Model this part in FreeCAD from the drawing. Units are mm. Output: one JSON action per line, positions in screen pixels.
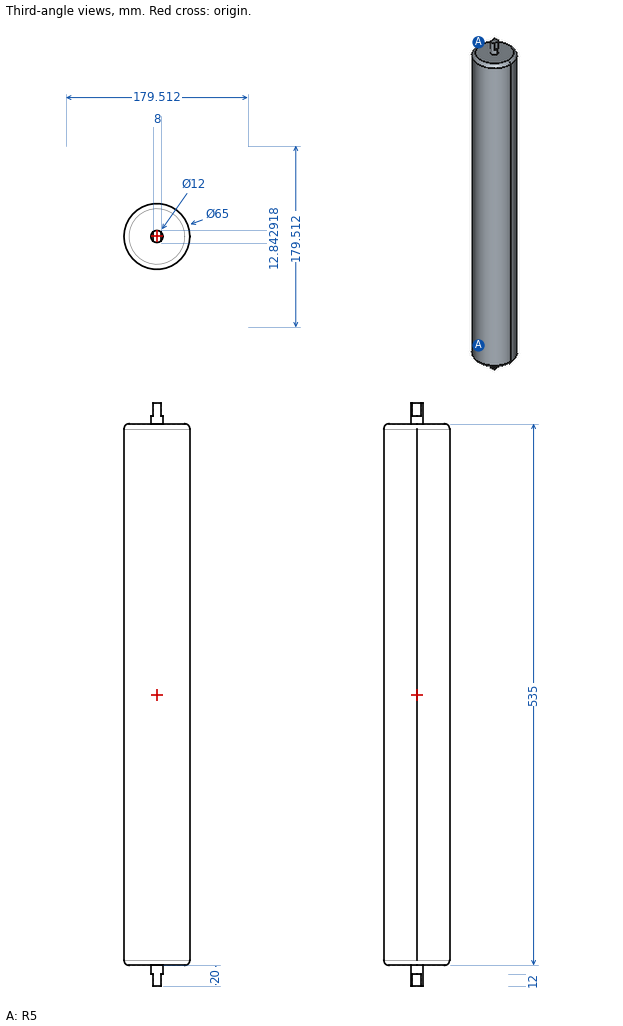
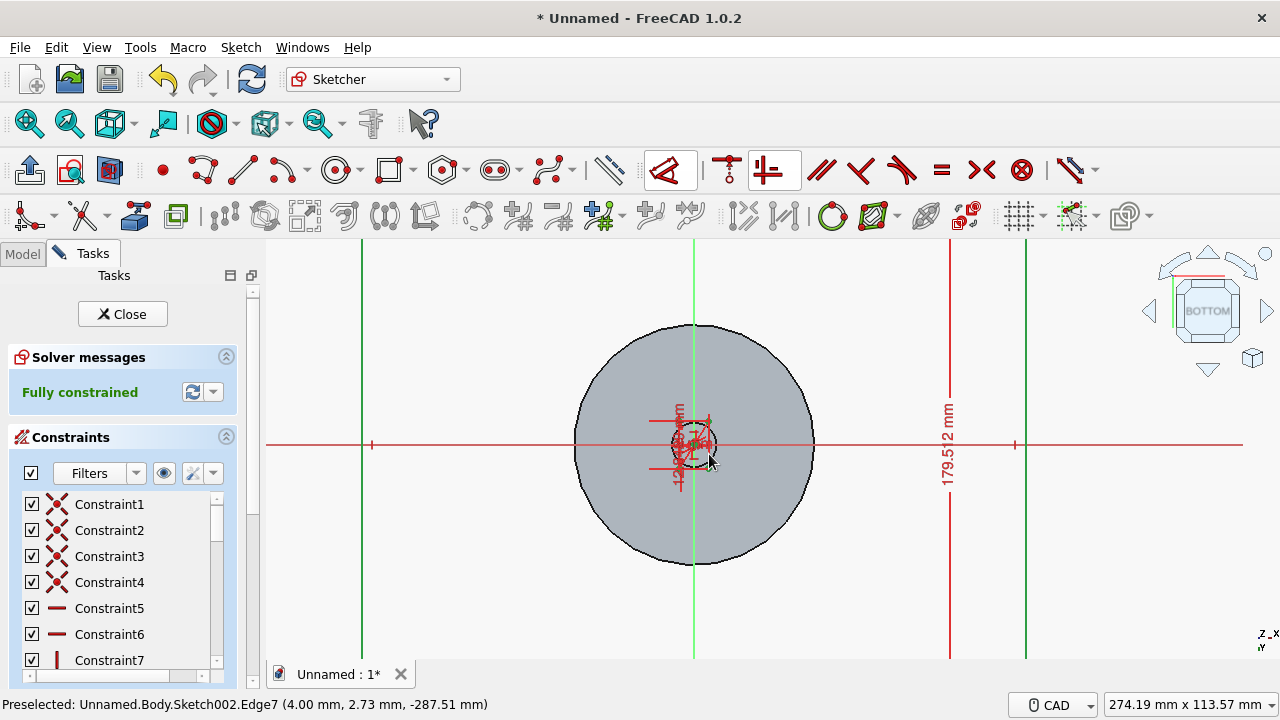
{"action": "left_click", "coordinate": [123, 314]}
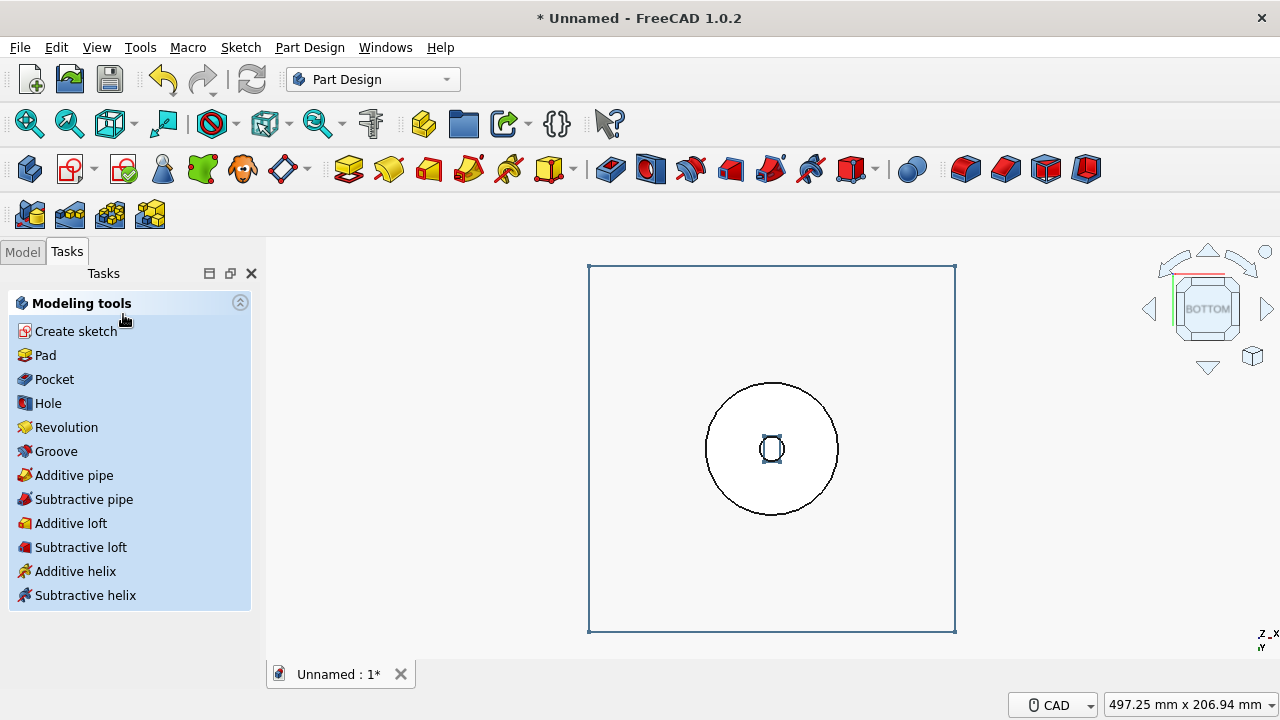
{"action": "left_click", "coordinate": [612, 170]}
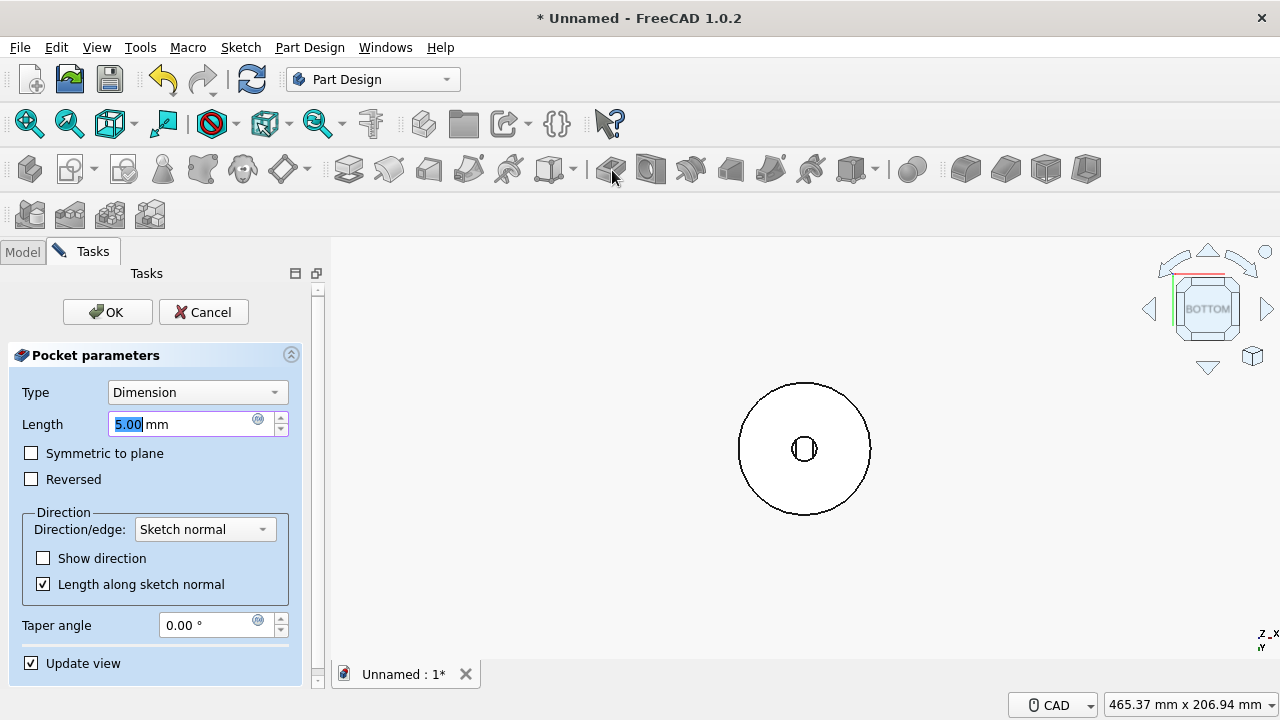
{"action": "type", "text": "12"}
{"action": "key", "text": "Tab"}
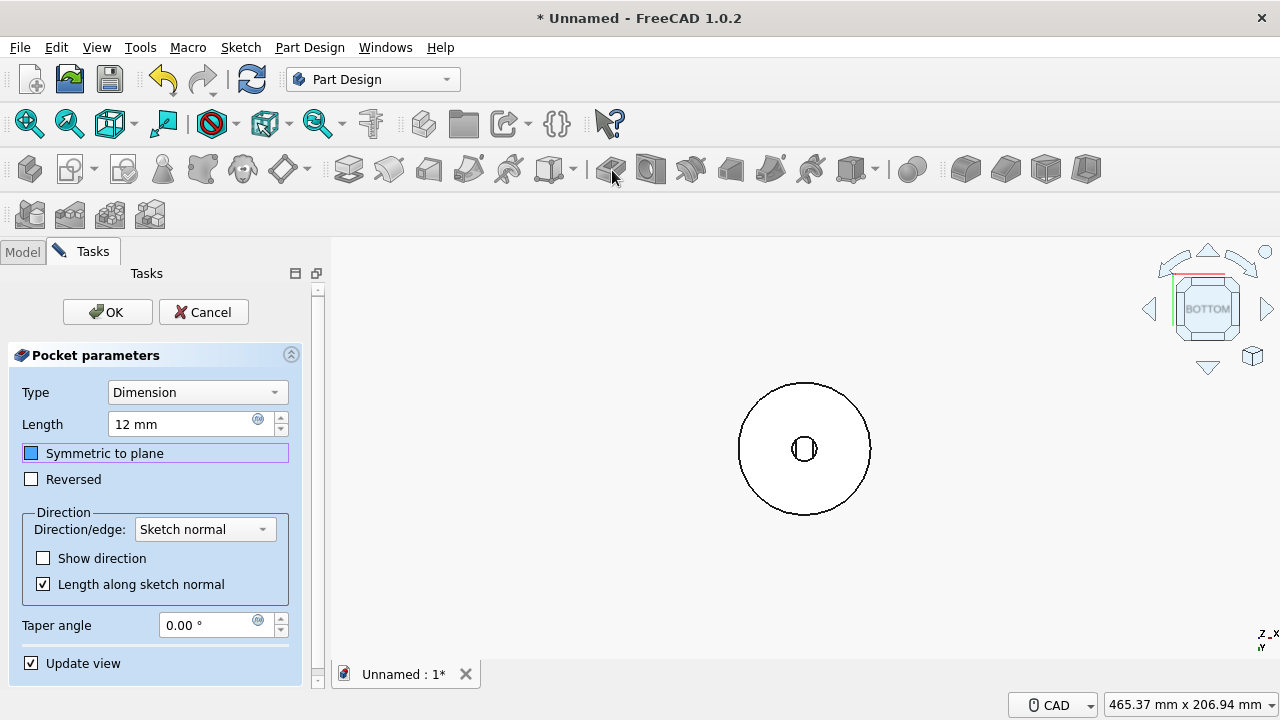
{"action": "left_click", "coordinate": [108, 312]}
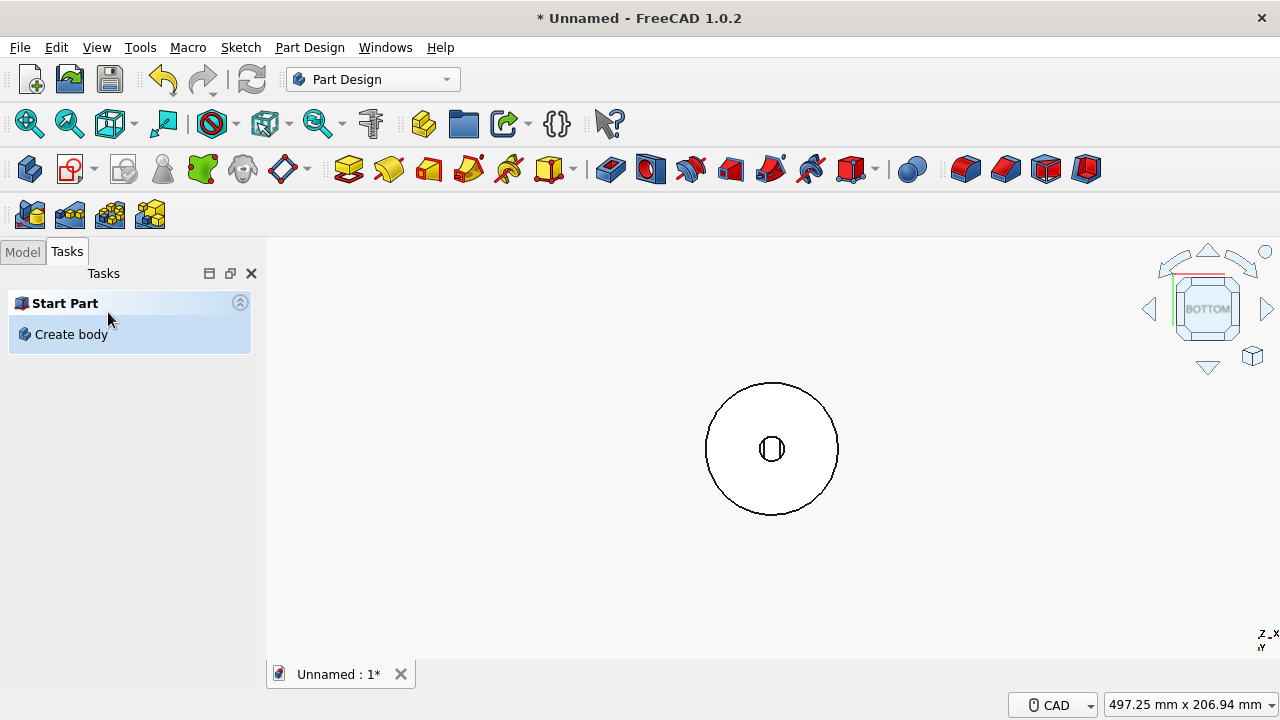
{"action": "left_click", "coordinate": [30, 124]}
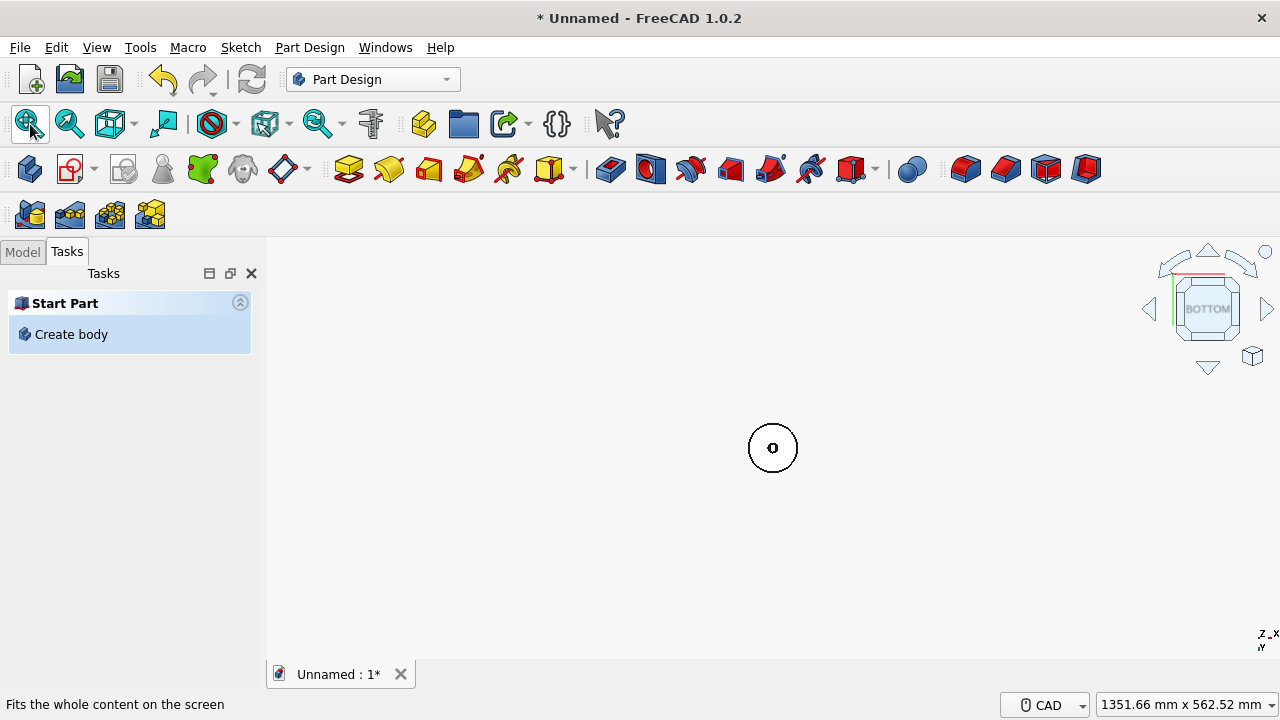
{"action": "left_click", "coordinate": [23, 251]}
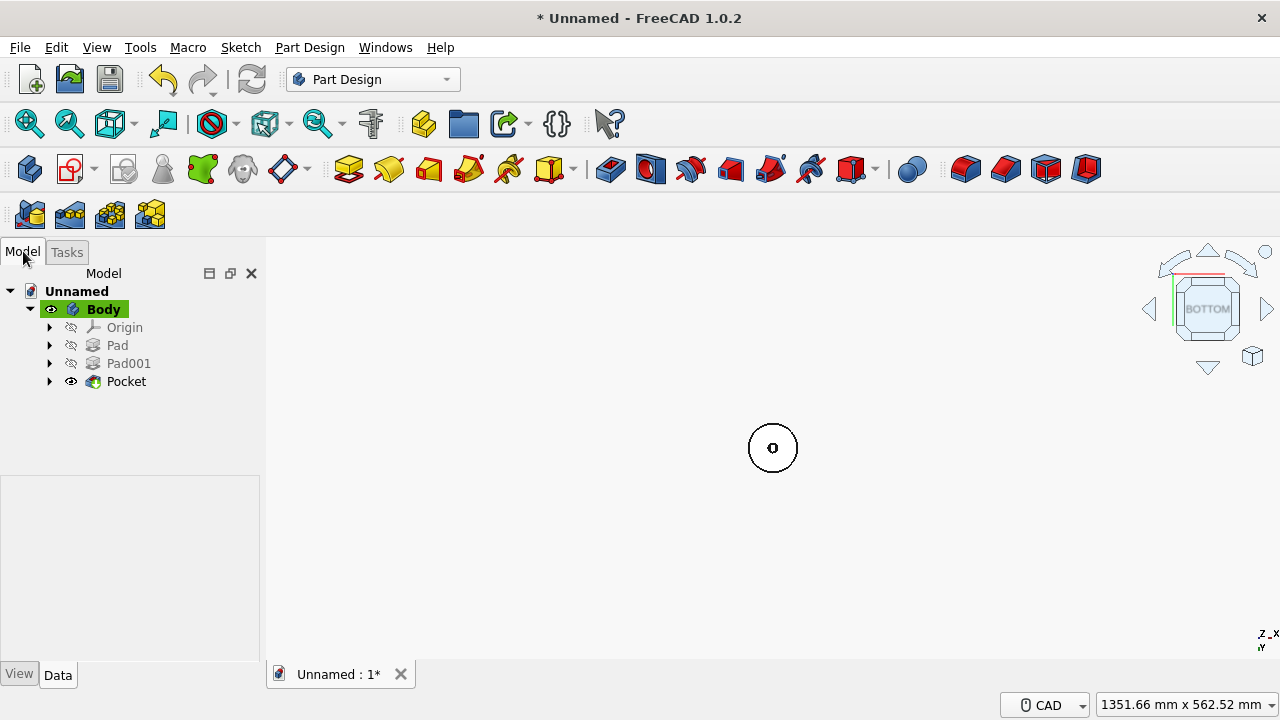
{"action": "left_click", "coordinate": [116, 363]}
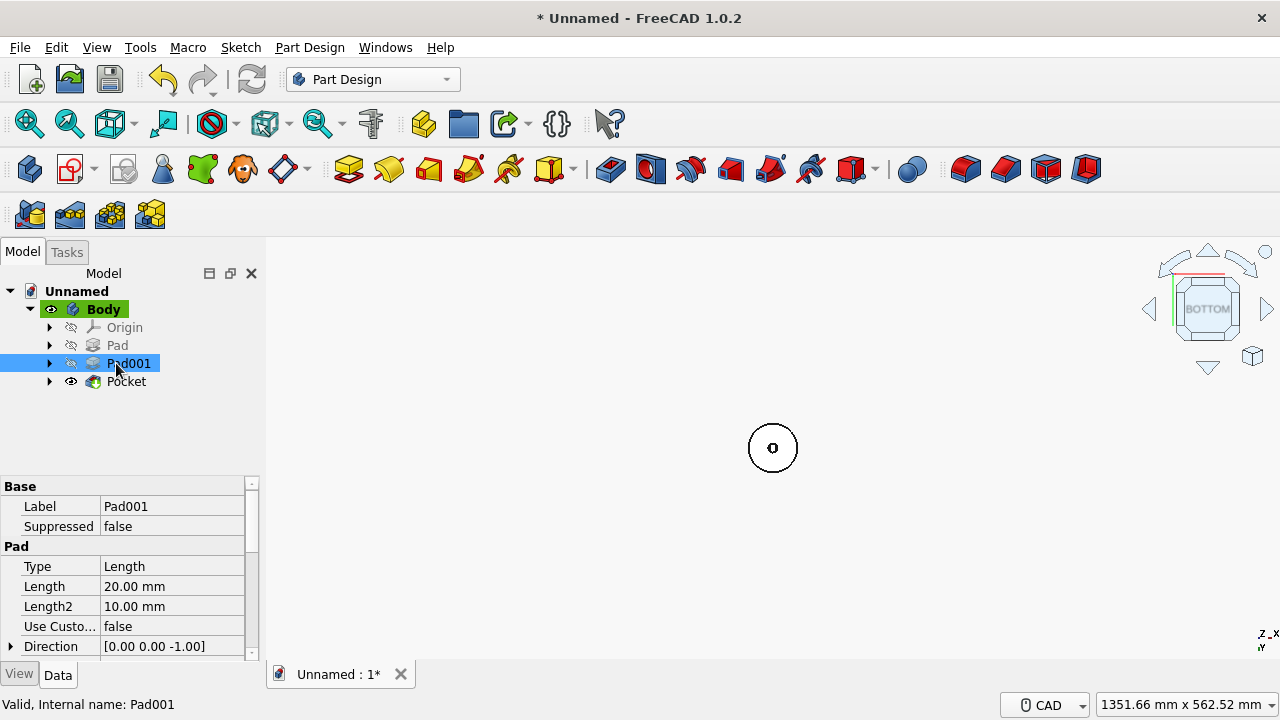
{"action": "left_click", "coordinate": [116, 381], "text": "ctrl"}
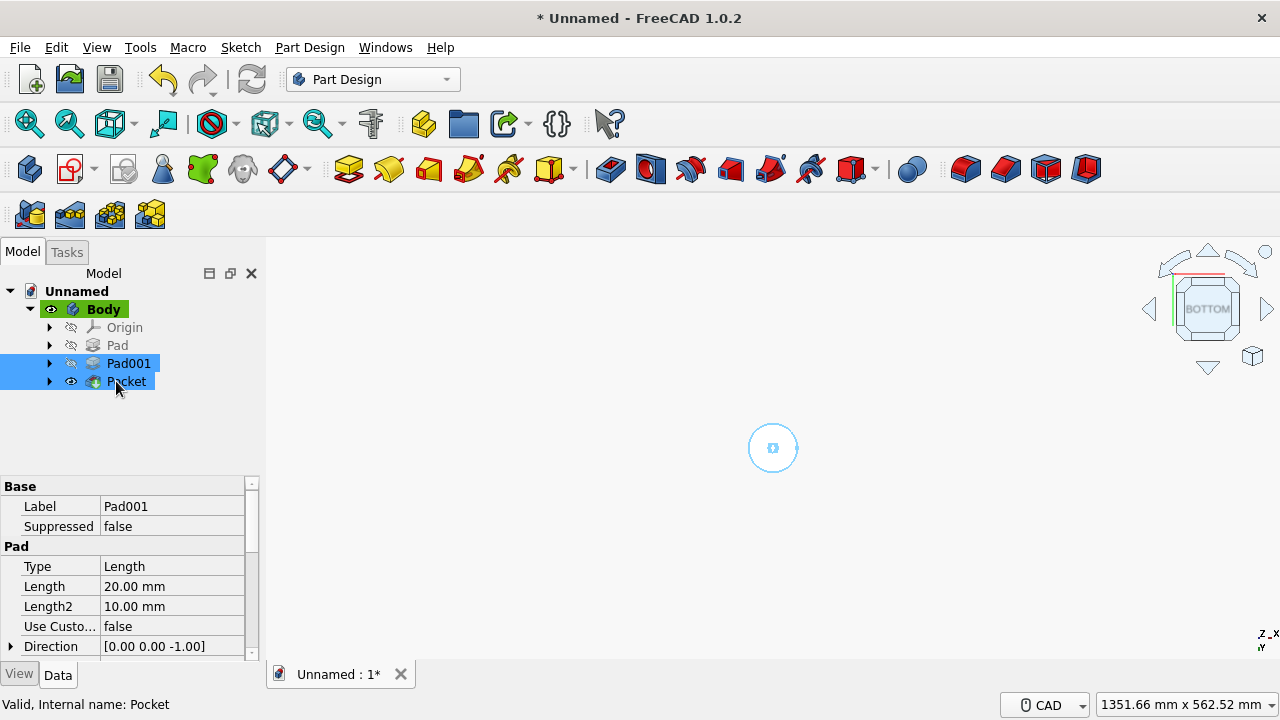
{"action": "left_click", "coordinate": [30, 214]}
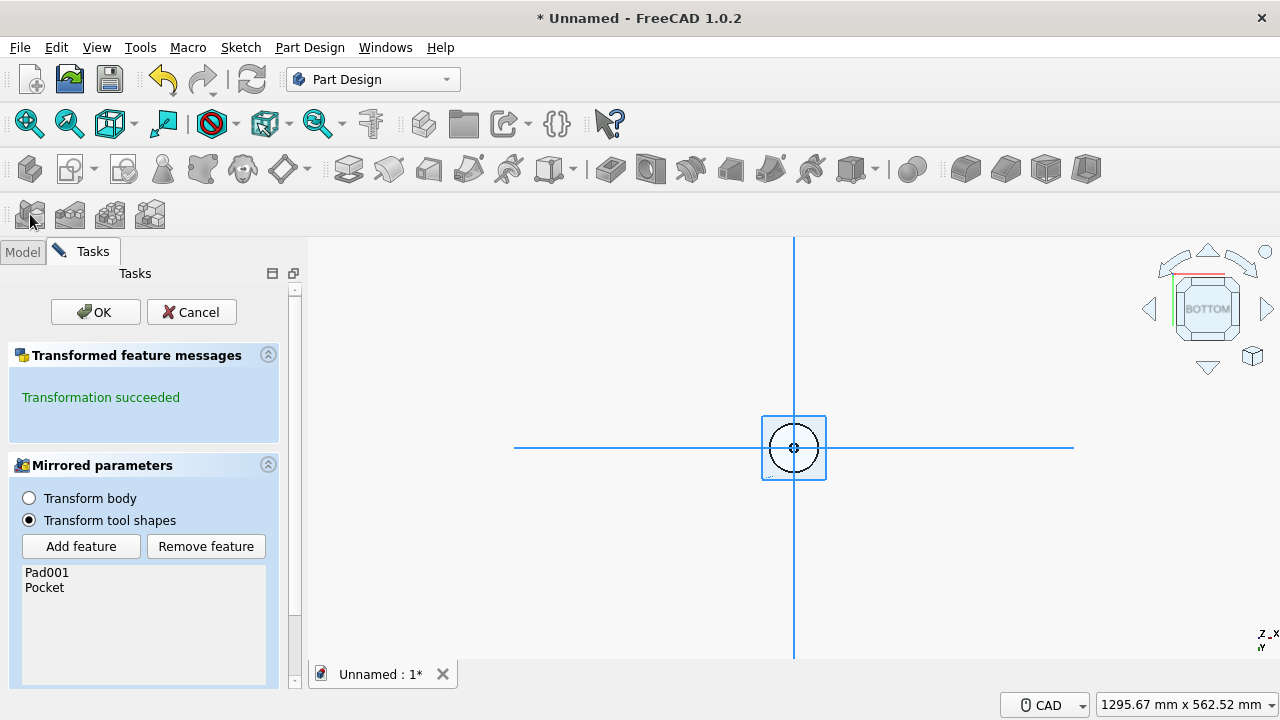
{"action": "scroll", "coordinate": [295, 486], "scroll_direction": "down", "scroll_amount": 2}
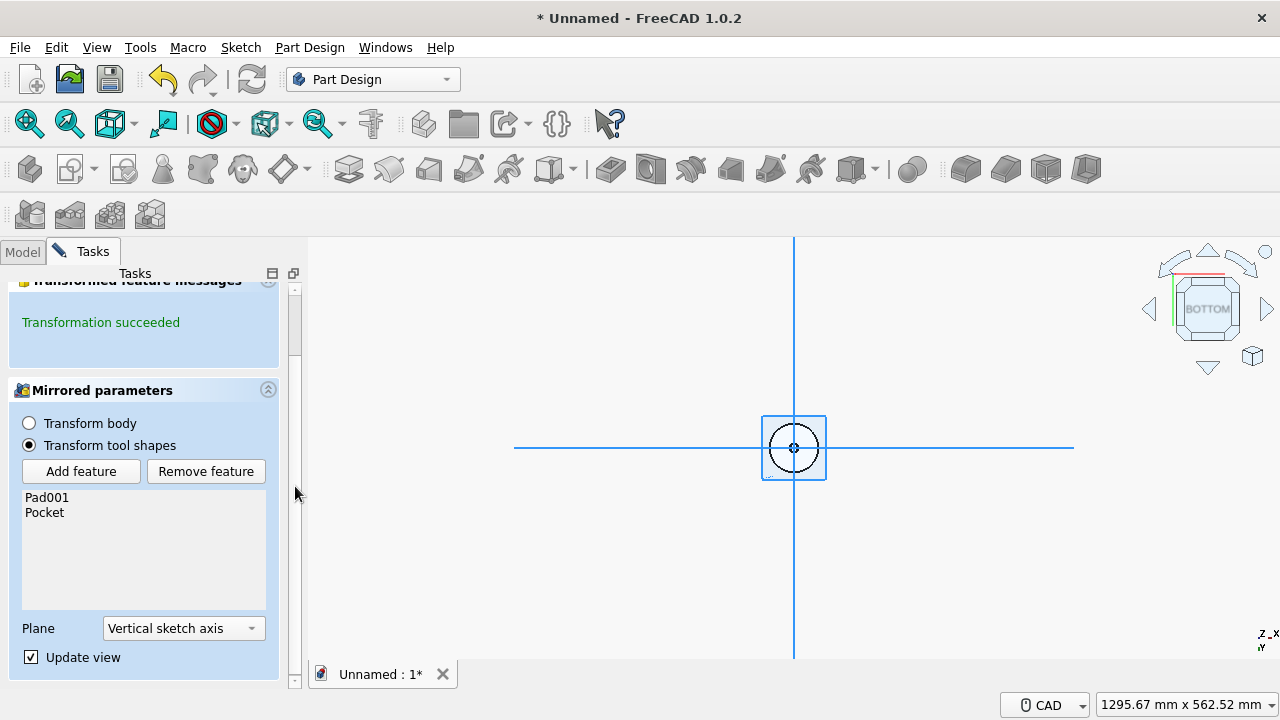
{"action": "left_click", "coordinate": [184, 628]}